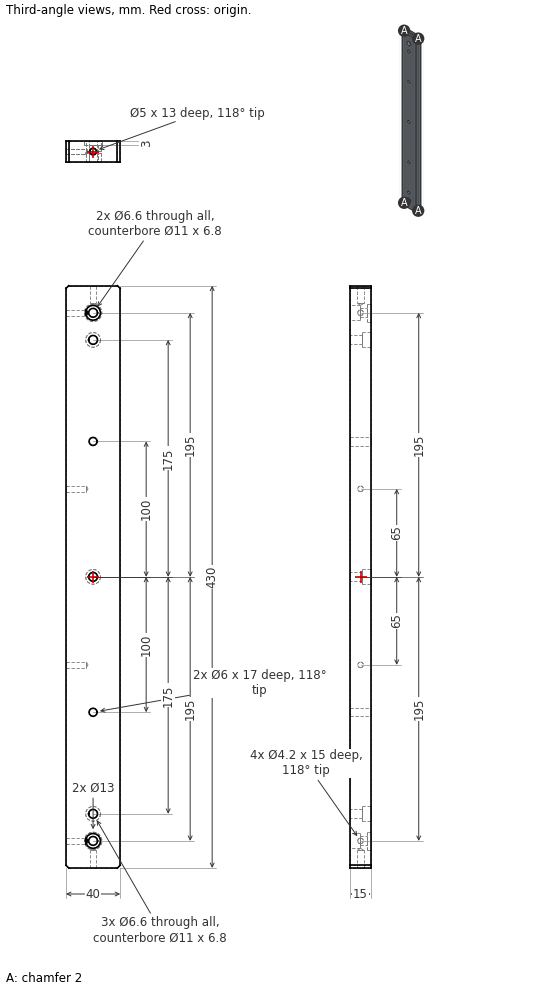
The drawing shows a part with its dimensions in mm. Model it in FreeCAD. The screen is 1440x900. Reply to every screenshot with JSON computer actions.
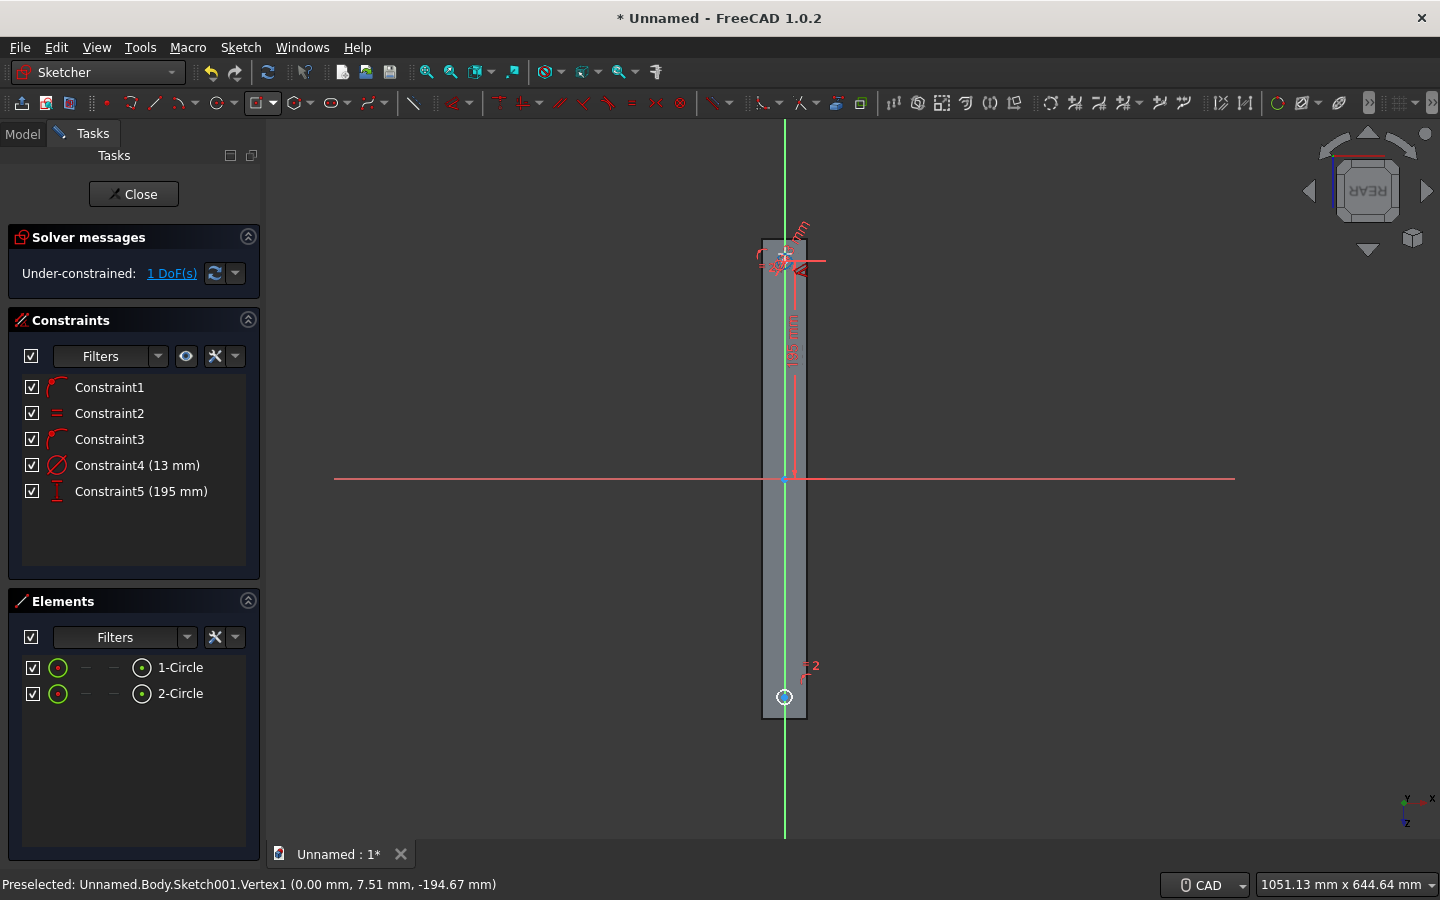
{"action": "left_click", "coordinate": [785, 697]}
{"action": "left_click", "coordinate": [819, 588]}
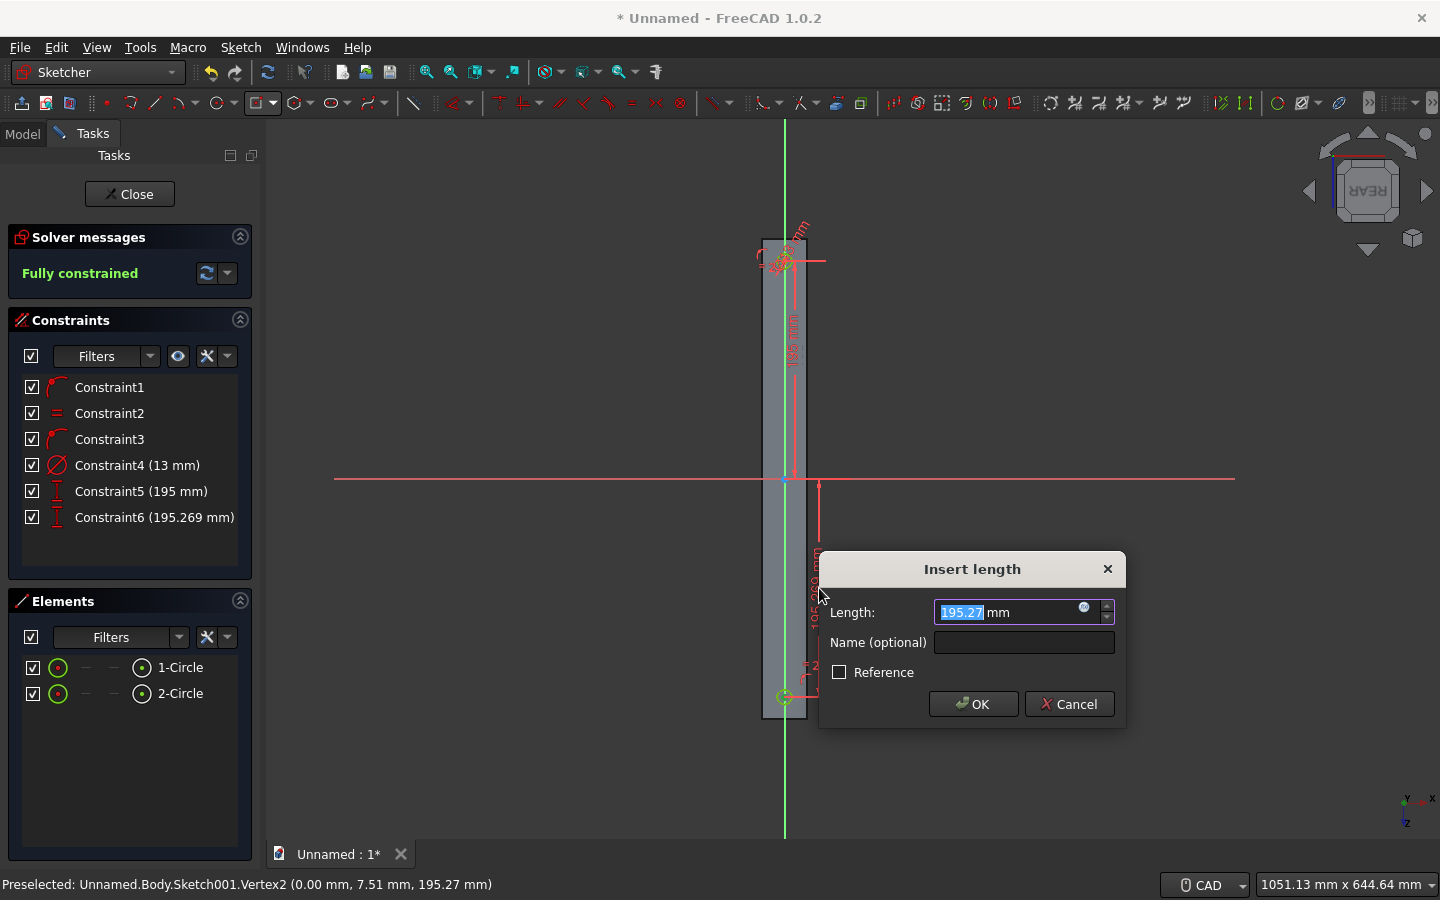
{"action": "type", "text": "195"}
{"action": "key", "text": "Return"}
{"action": "key", "text": "Escape"}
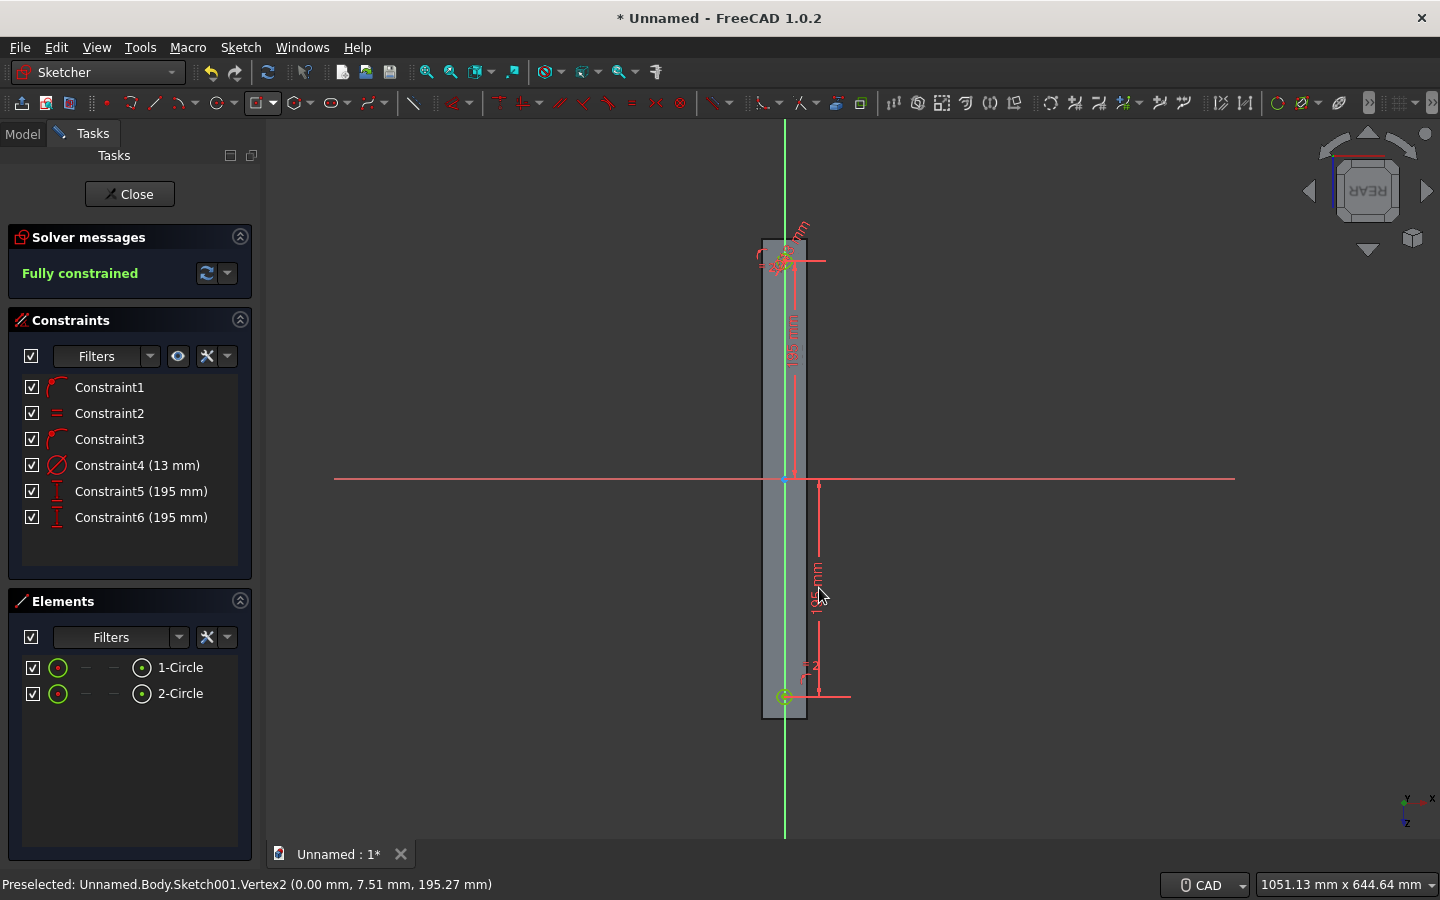
{"action": "left_click", "coordinate": [130, 194]}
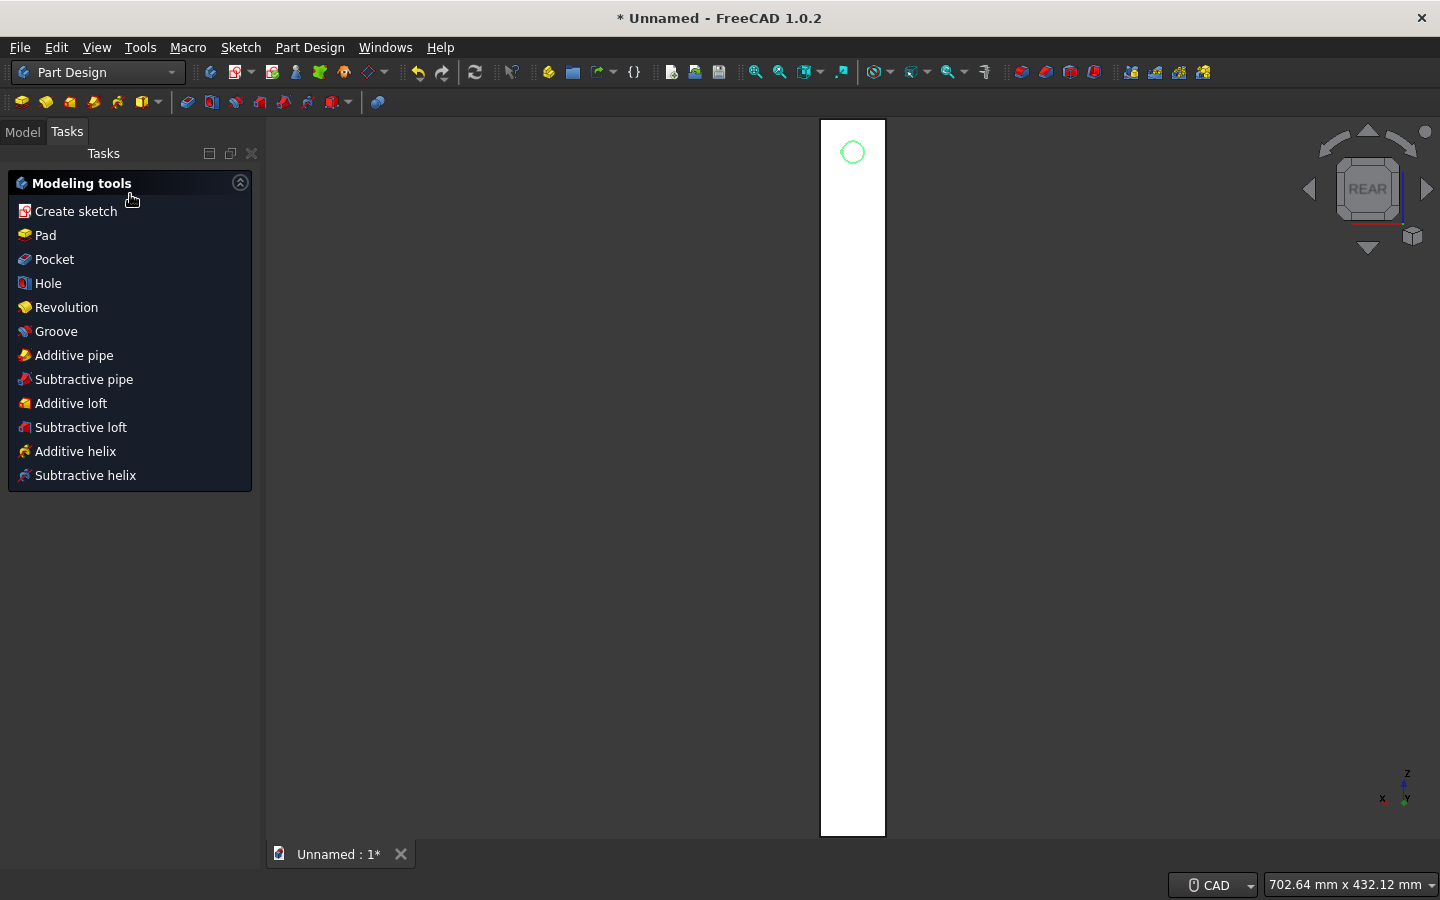
{"action": "left_click", "coordinate": [188, 102]}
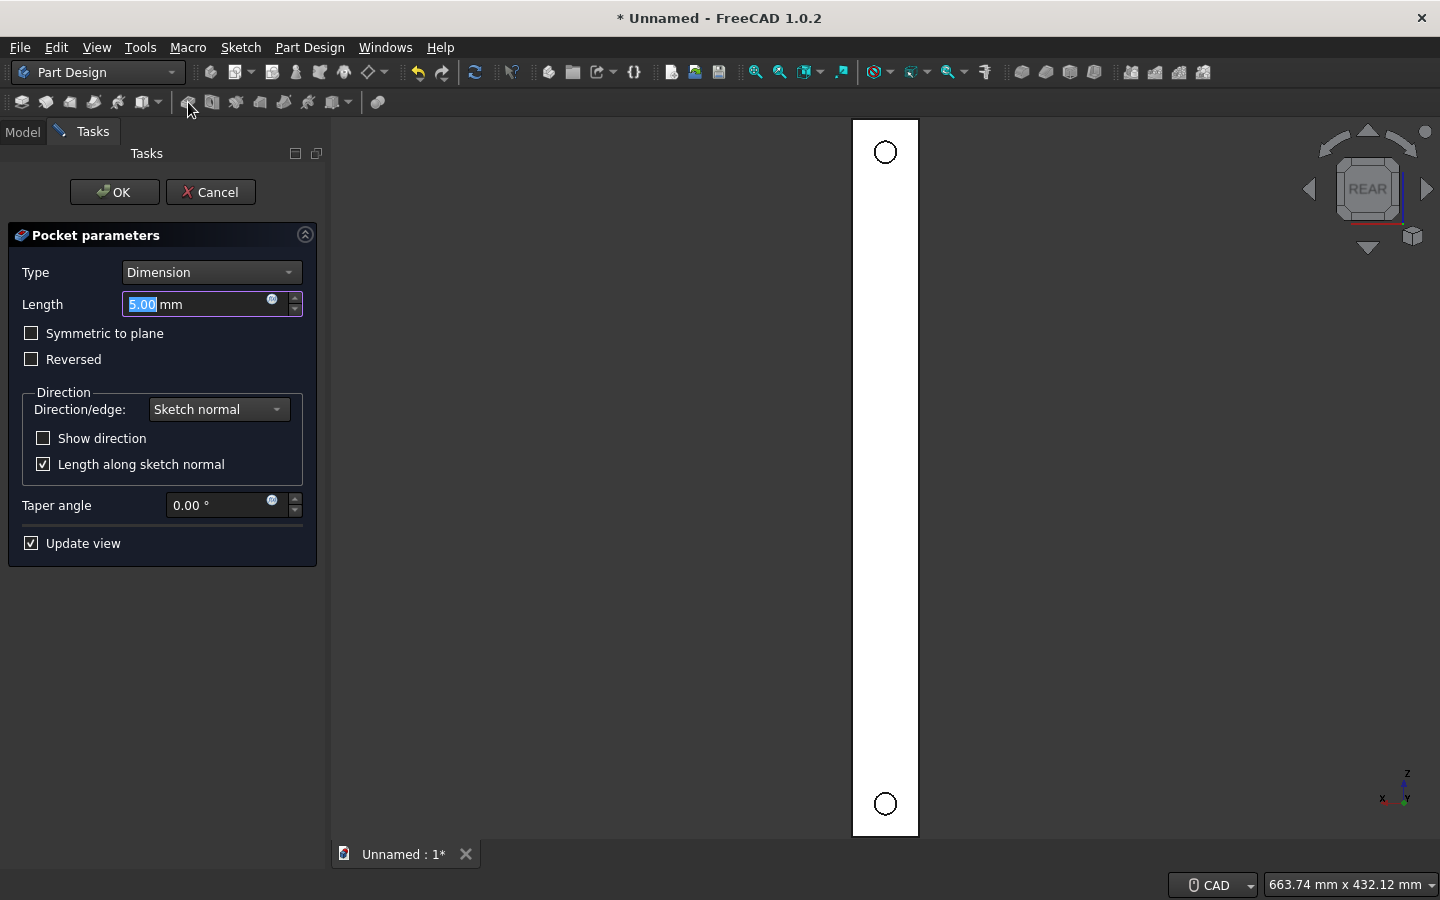
{"action": "type", "text": "3"}
{"action": "key", "text": "Tab"}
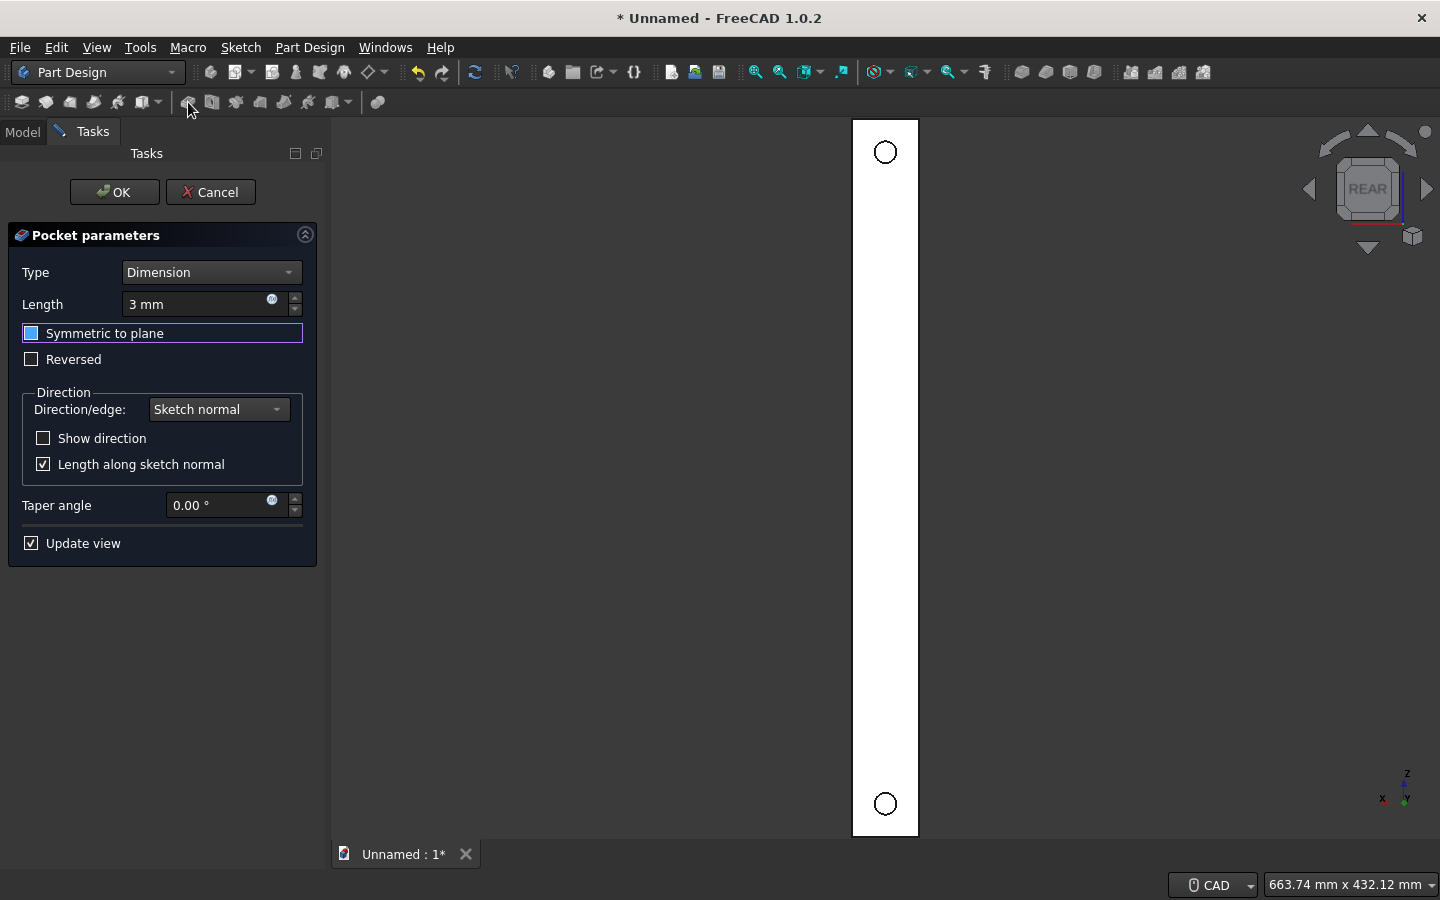
{"action": "left_click", "coordinate": [115, 192]}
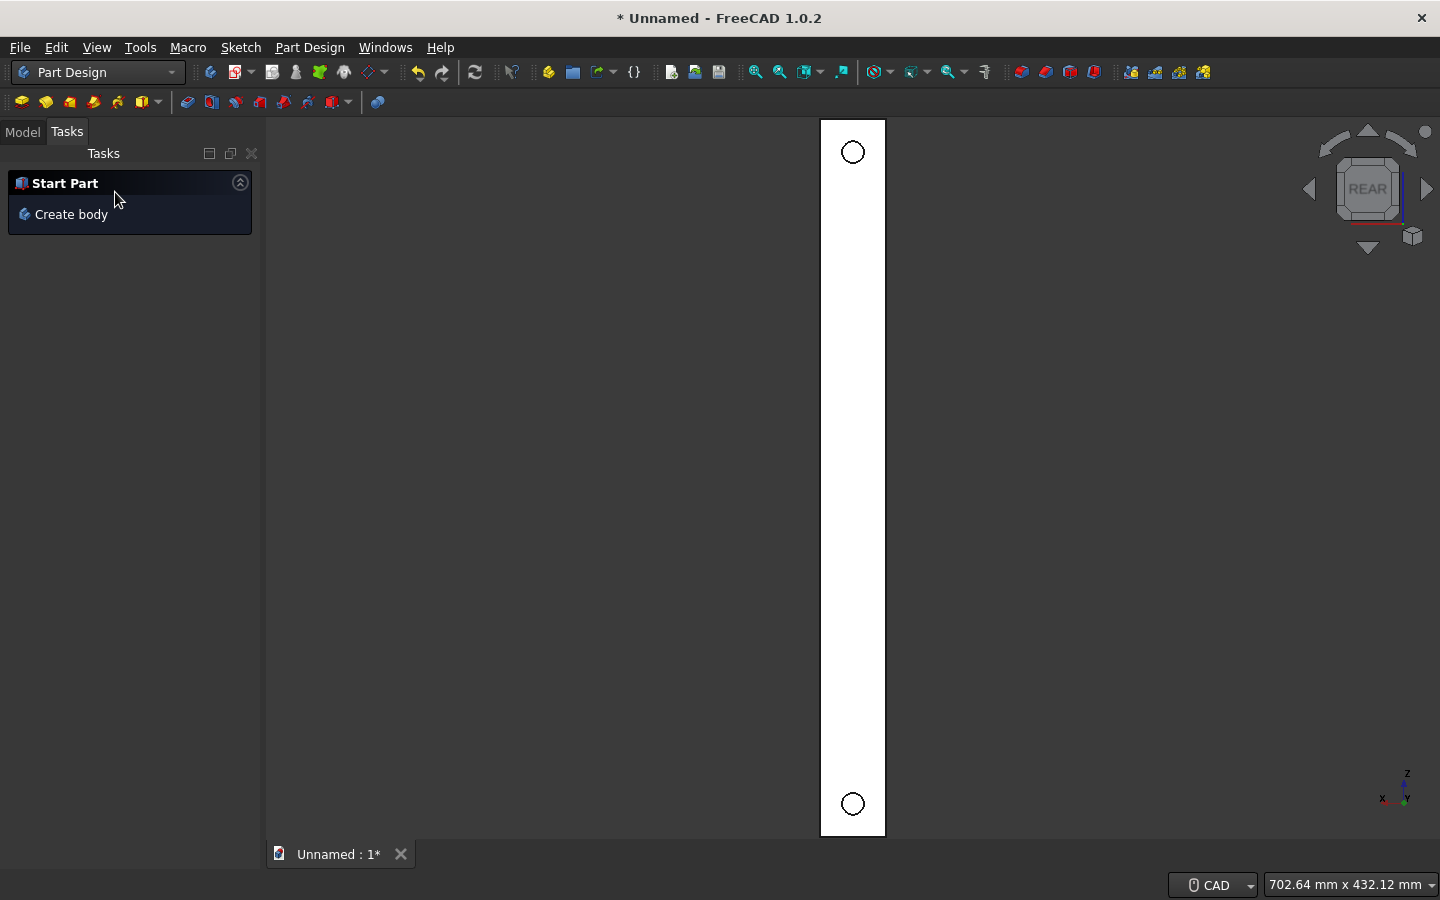
{"action": "key", "text": "0"}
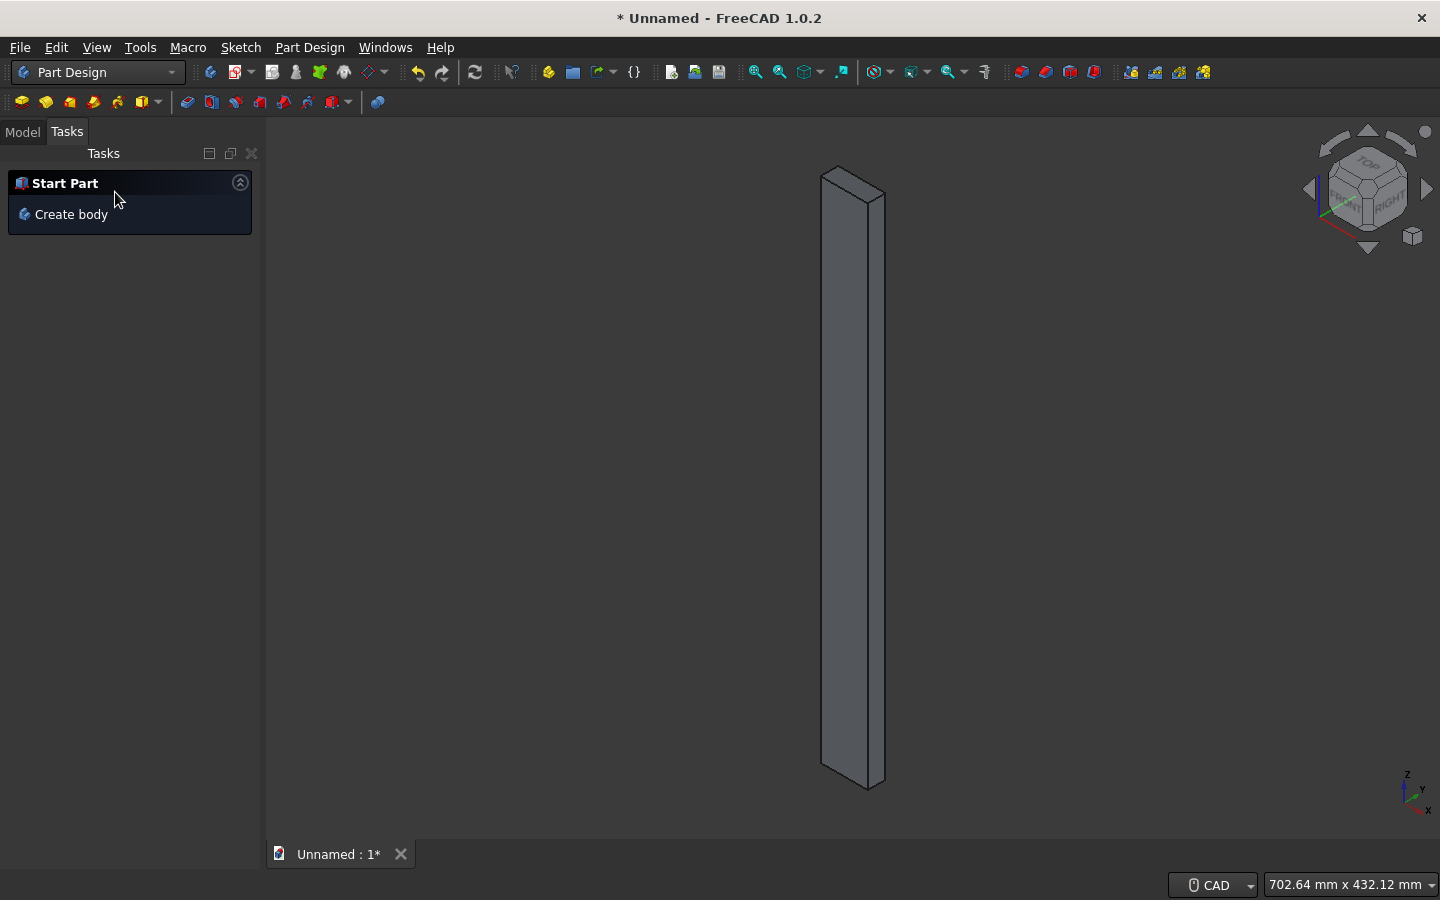
{"action": "left_click", "coordinate": [844, 231]}